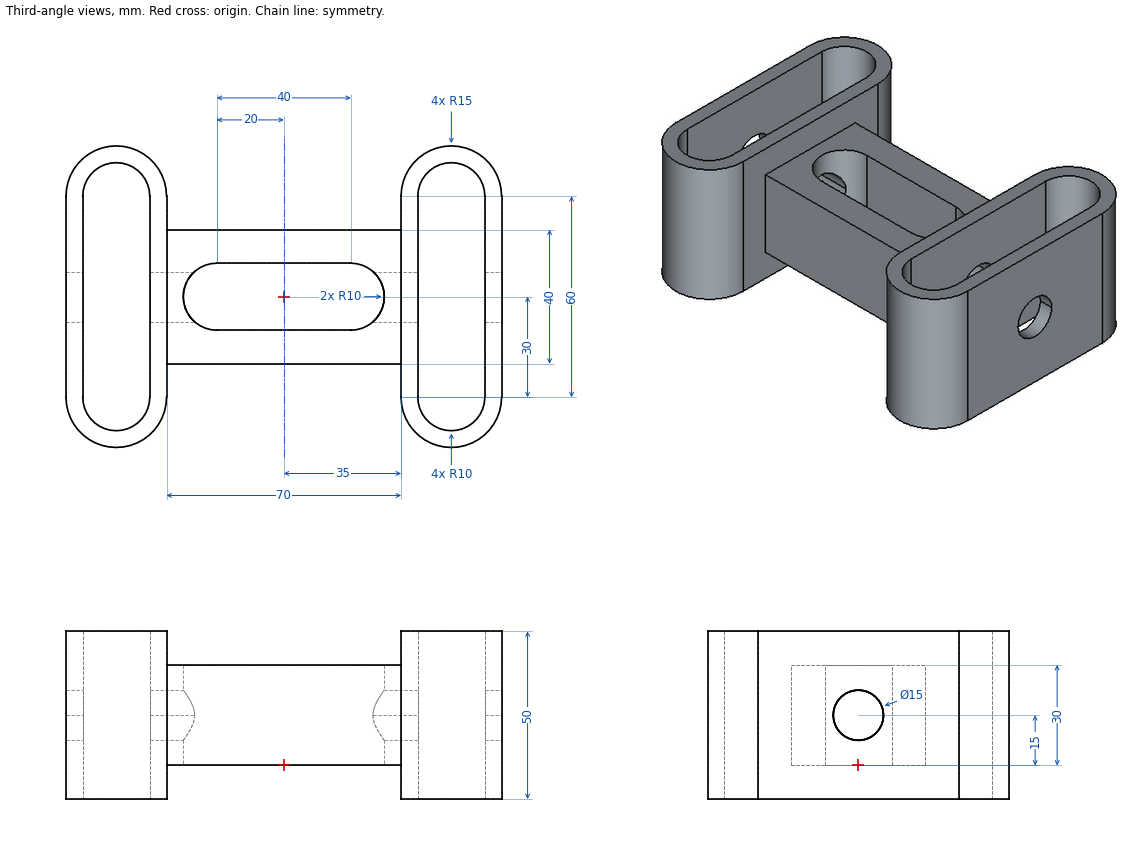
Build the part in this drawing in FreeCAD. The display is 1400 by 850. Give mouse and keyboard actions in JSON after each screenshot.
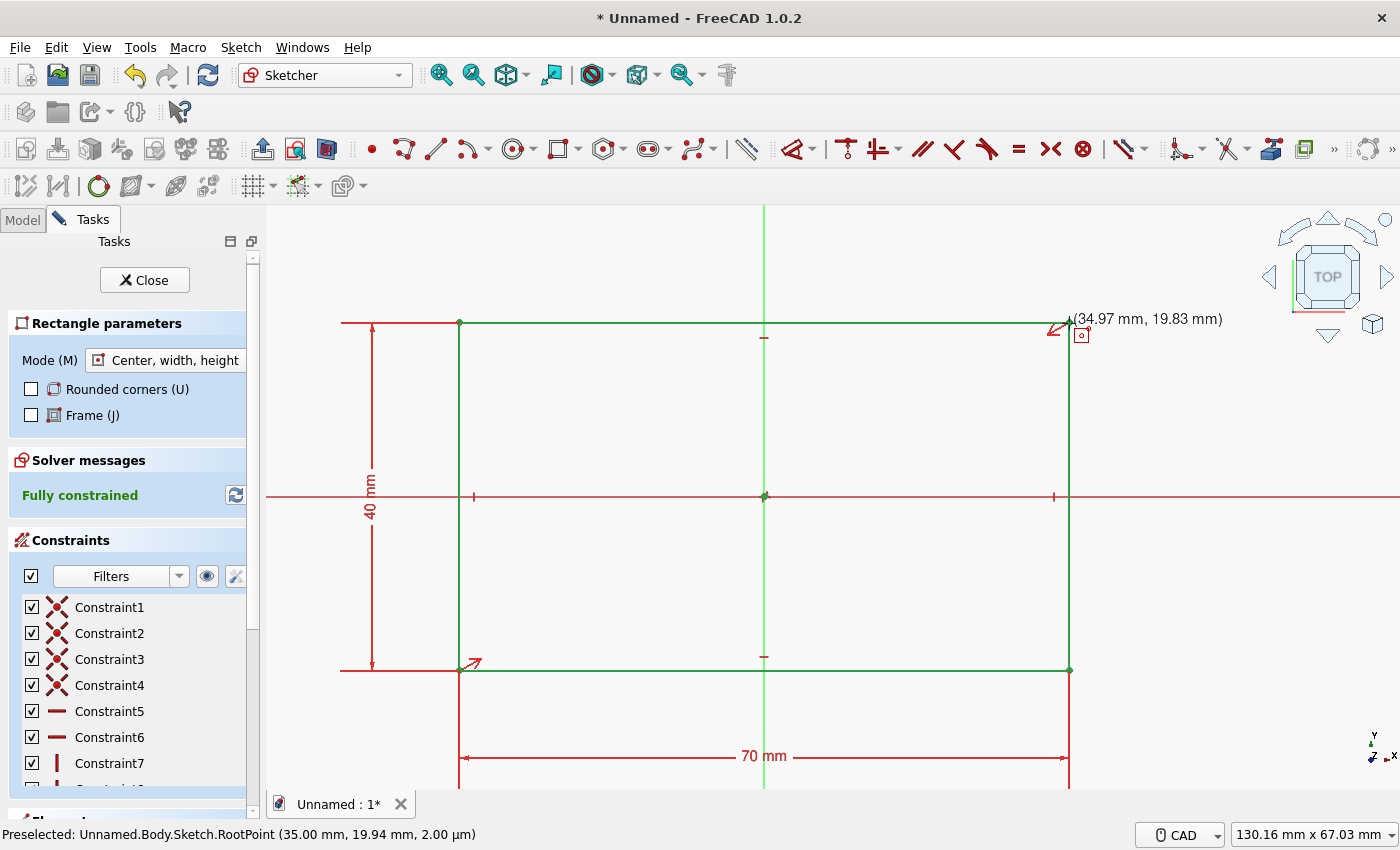
{"action": "key", "text": "g s"}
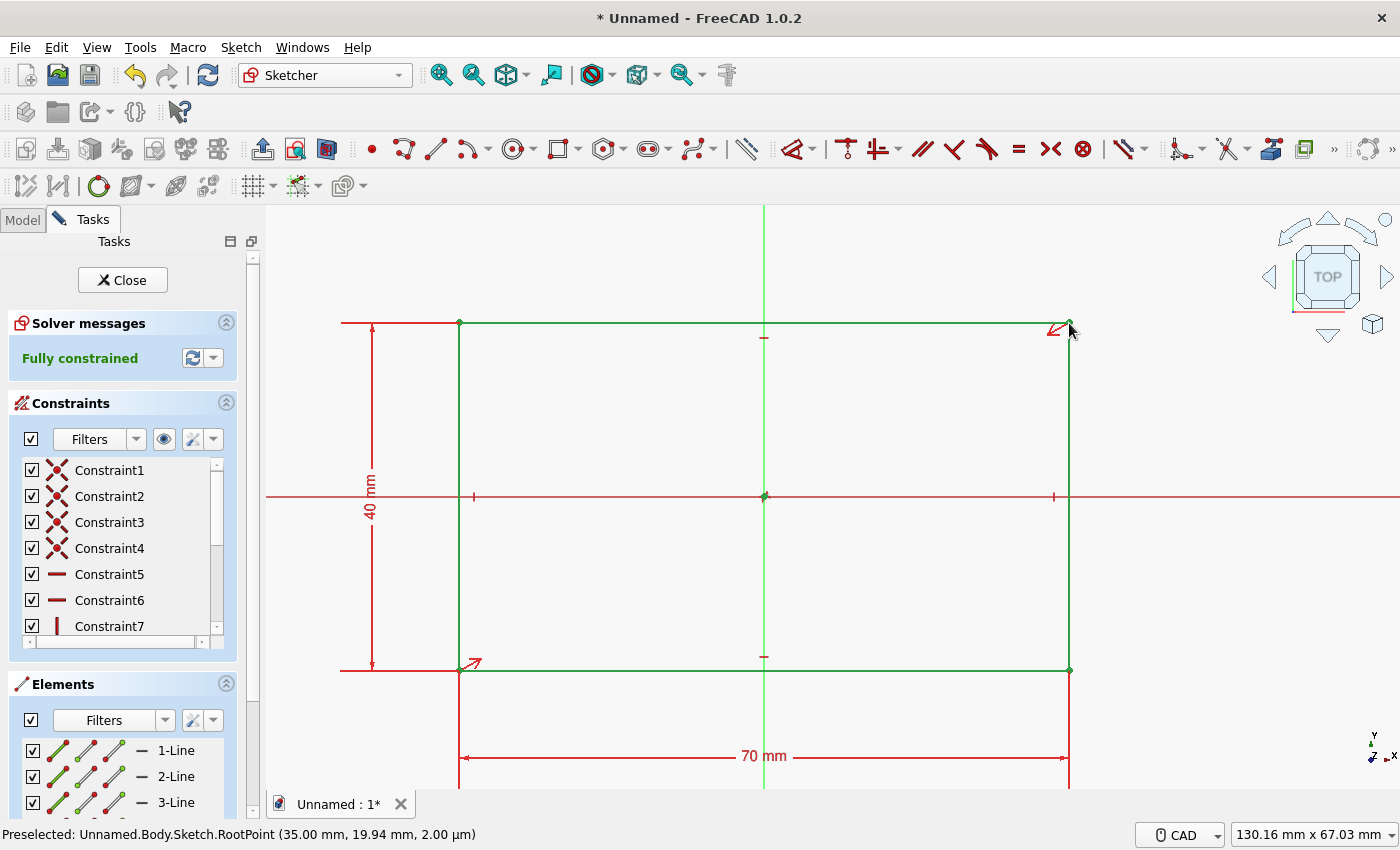
{"action": "left_click", "coordinate": [590, 497]}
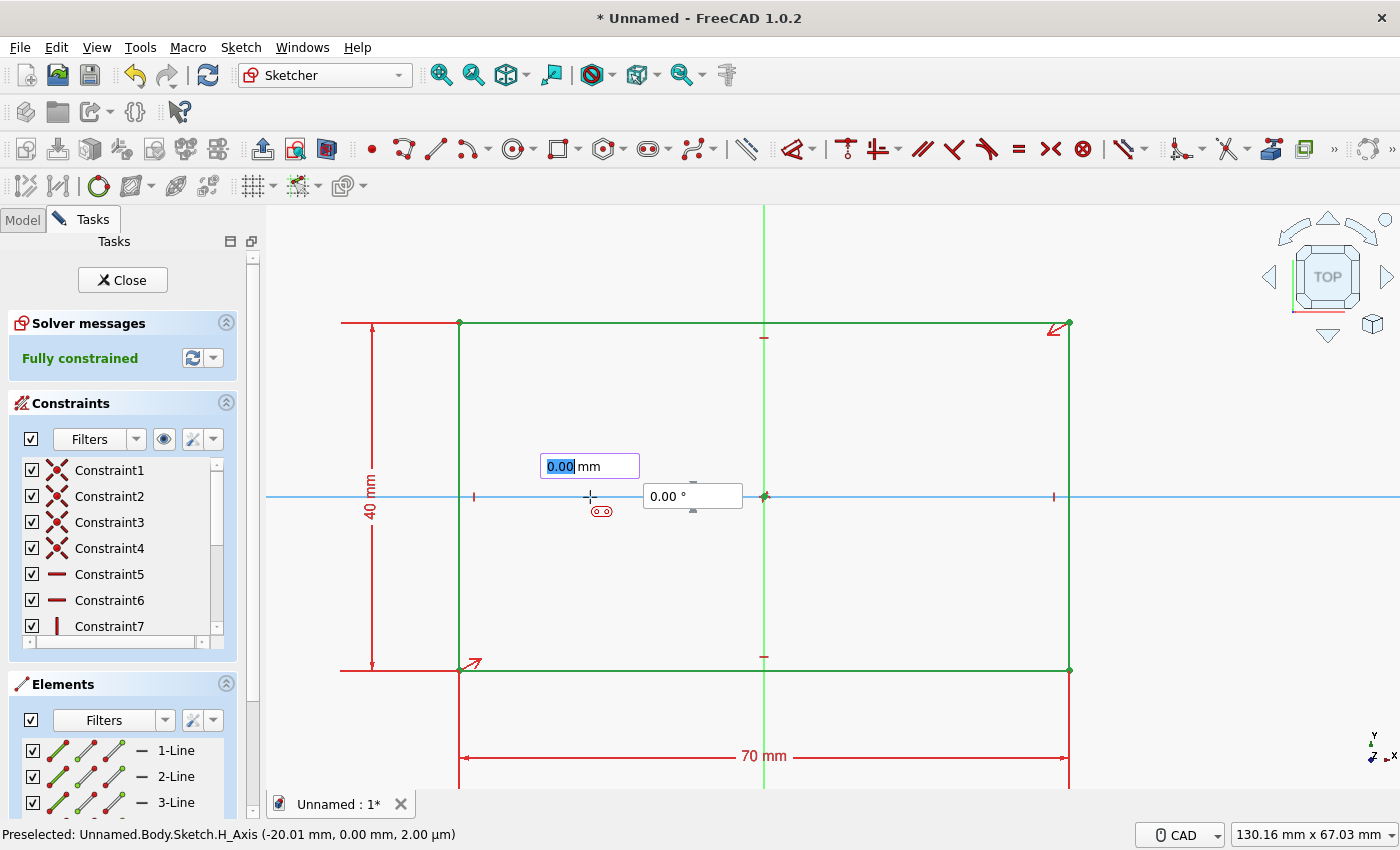
{"action": "left_click", "coordinate": [939, 488]}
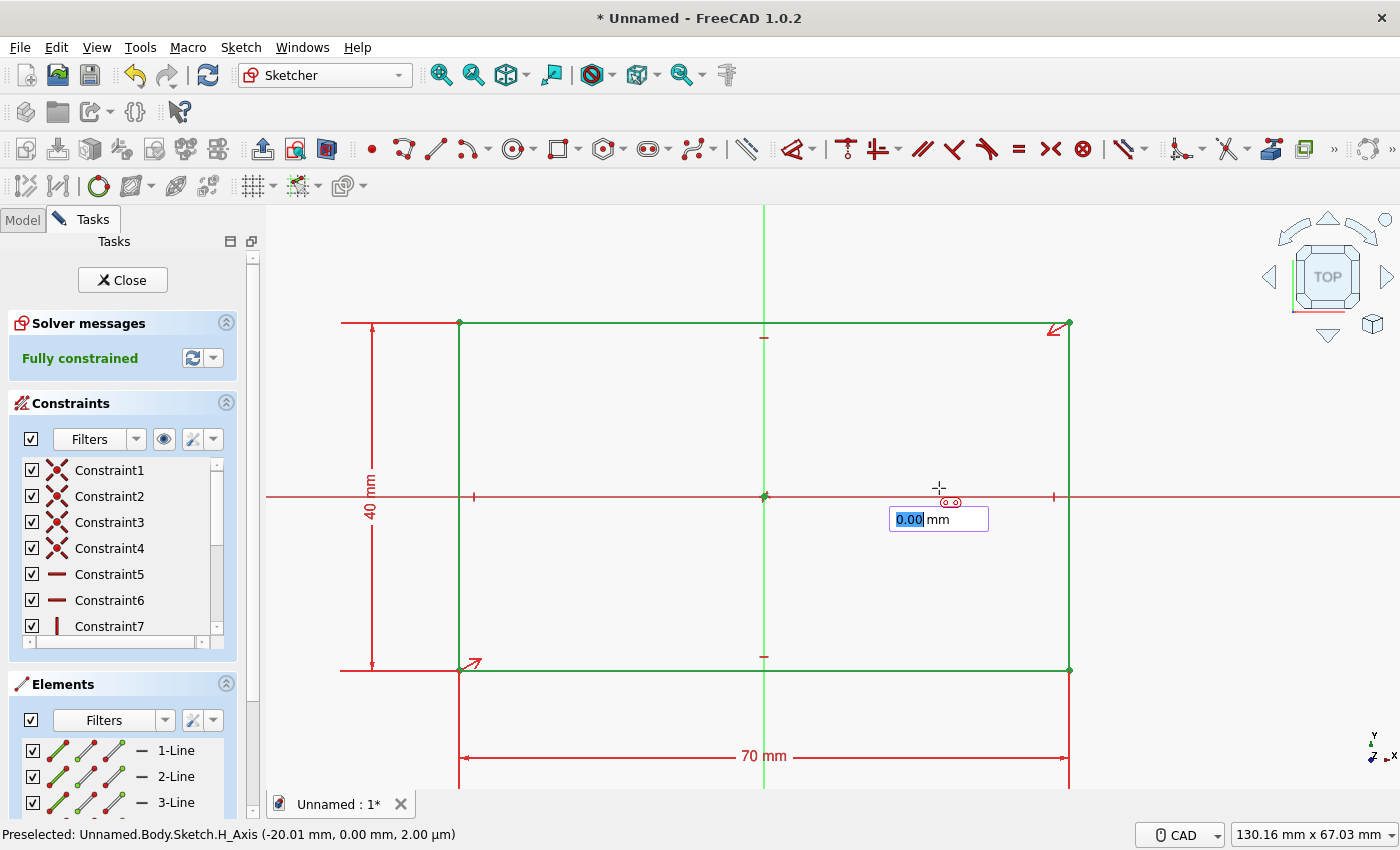
{"action": "left_click", "coordinate": [817, 584]}
{"action": "key", "text": "Escape"}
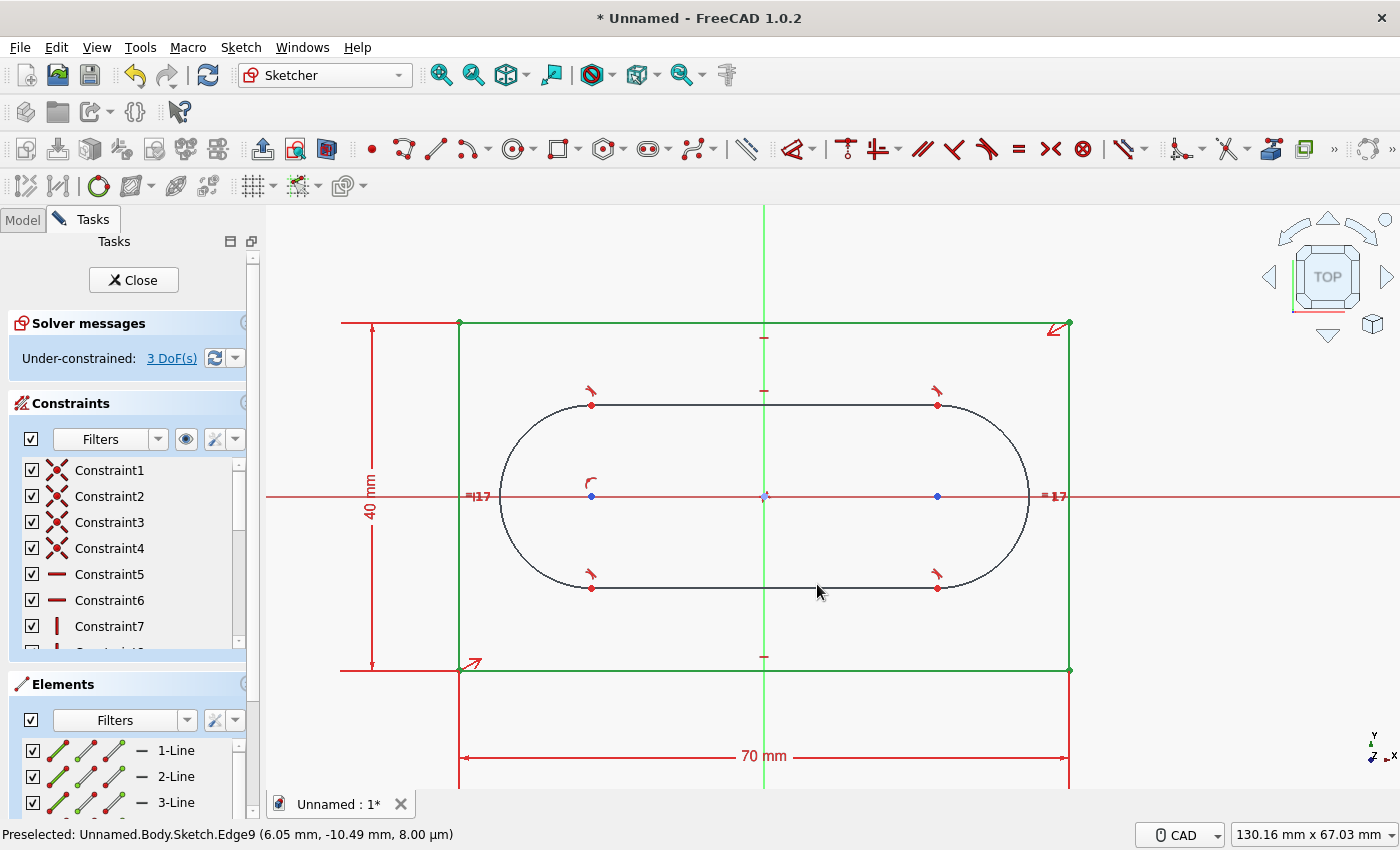
{"action": "left_click", "coordinate": [792, 150]}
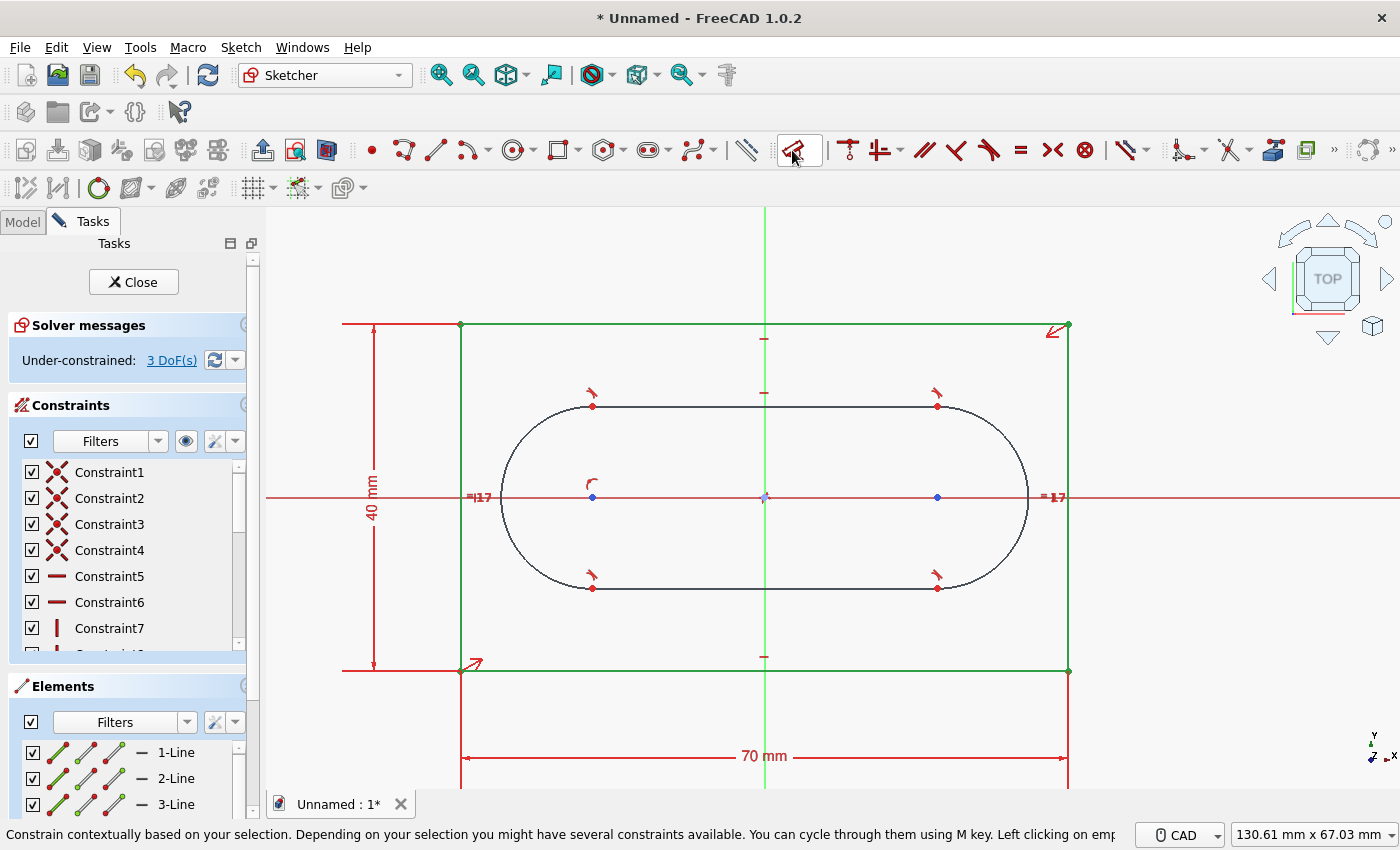
{"action": "left_click", "coordinate": [519, 444]}
{"action": "left_click", "coordinate": [493, 425]}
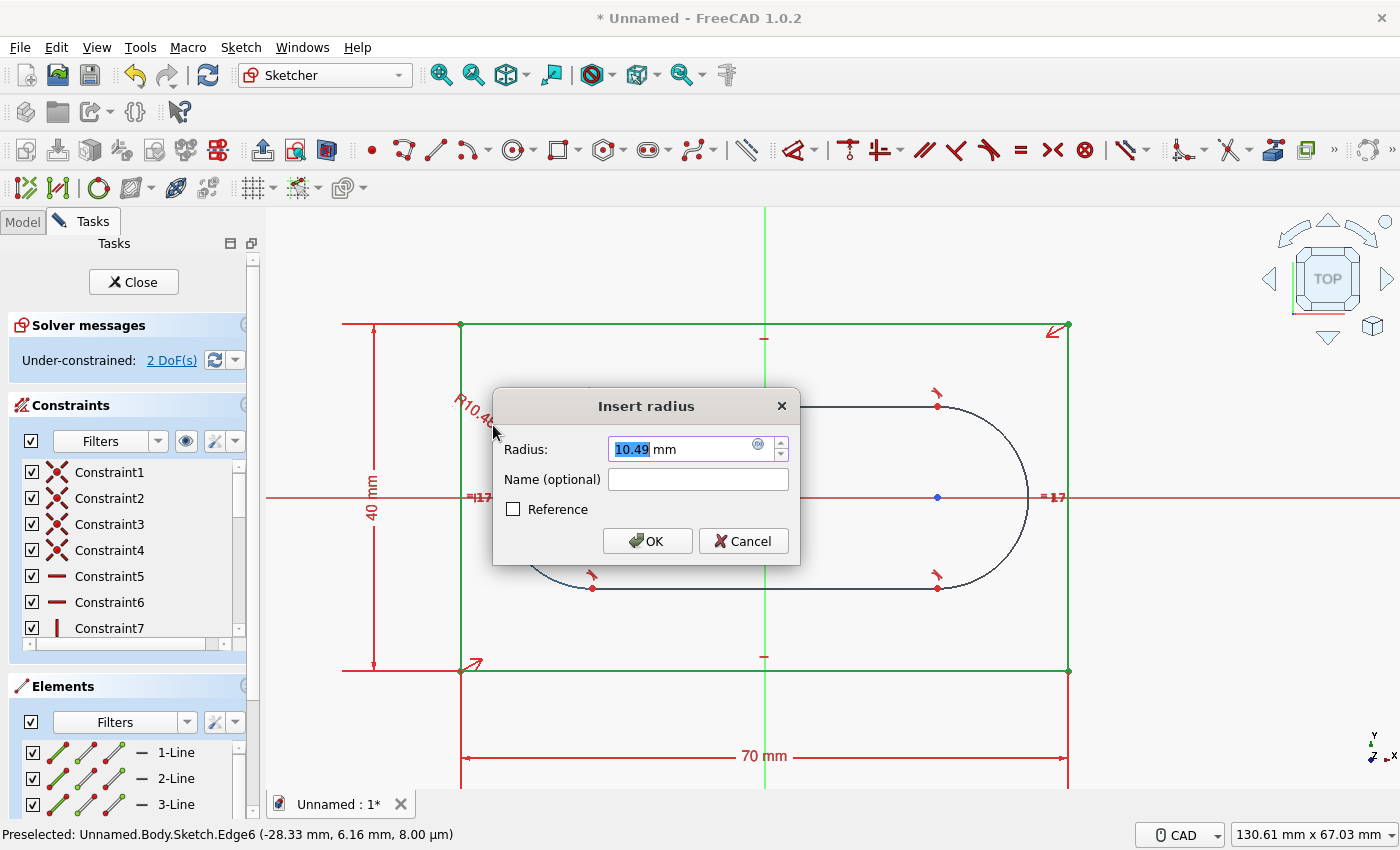
{"action": "type", "text": "10"}
{"action": "key", "text": "Return"}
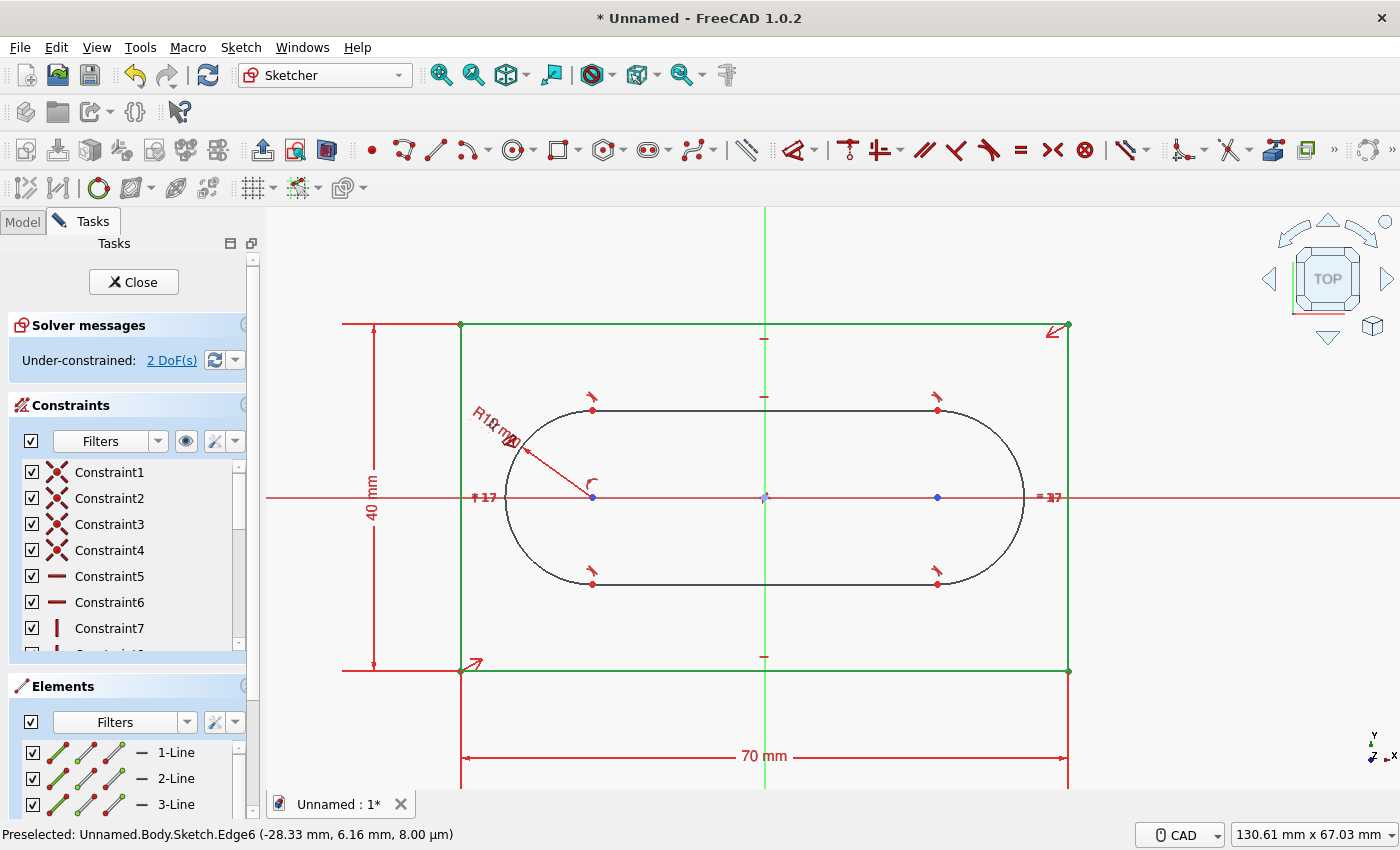
{"action": "left_click", "coordinate": [696, 411]}
{"action": "left_click", "coordinate": [685, 377]}